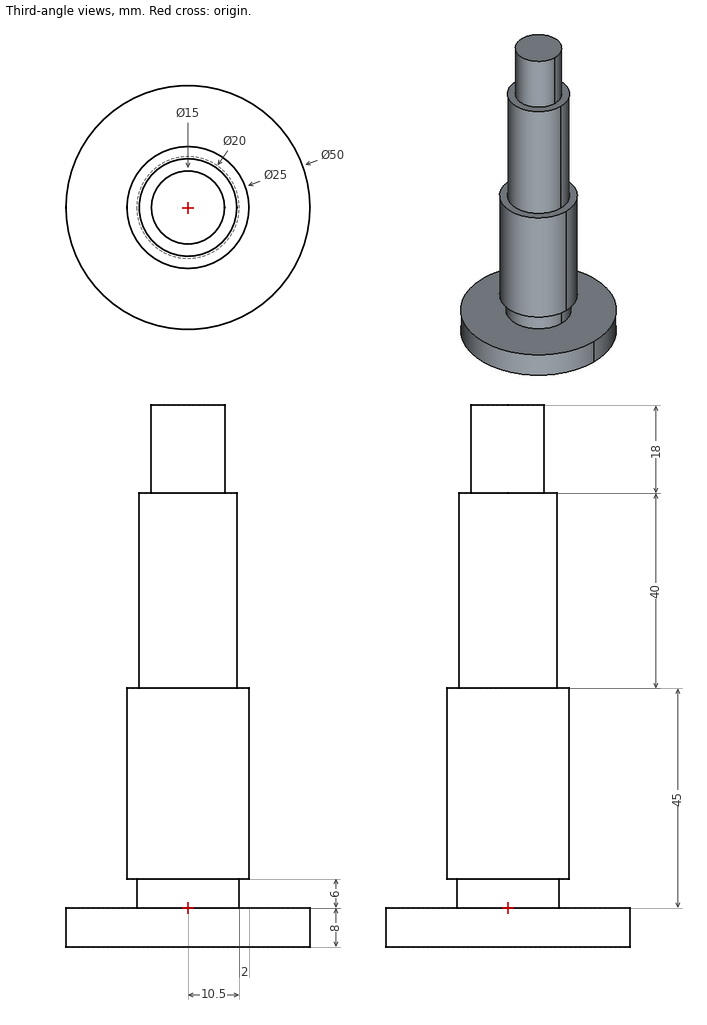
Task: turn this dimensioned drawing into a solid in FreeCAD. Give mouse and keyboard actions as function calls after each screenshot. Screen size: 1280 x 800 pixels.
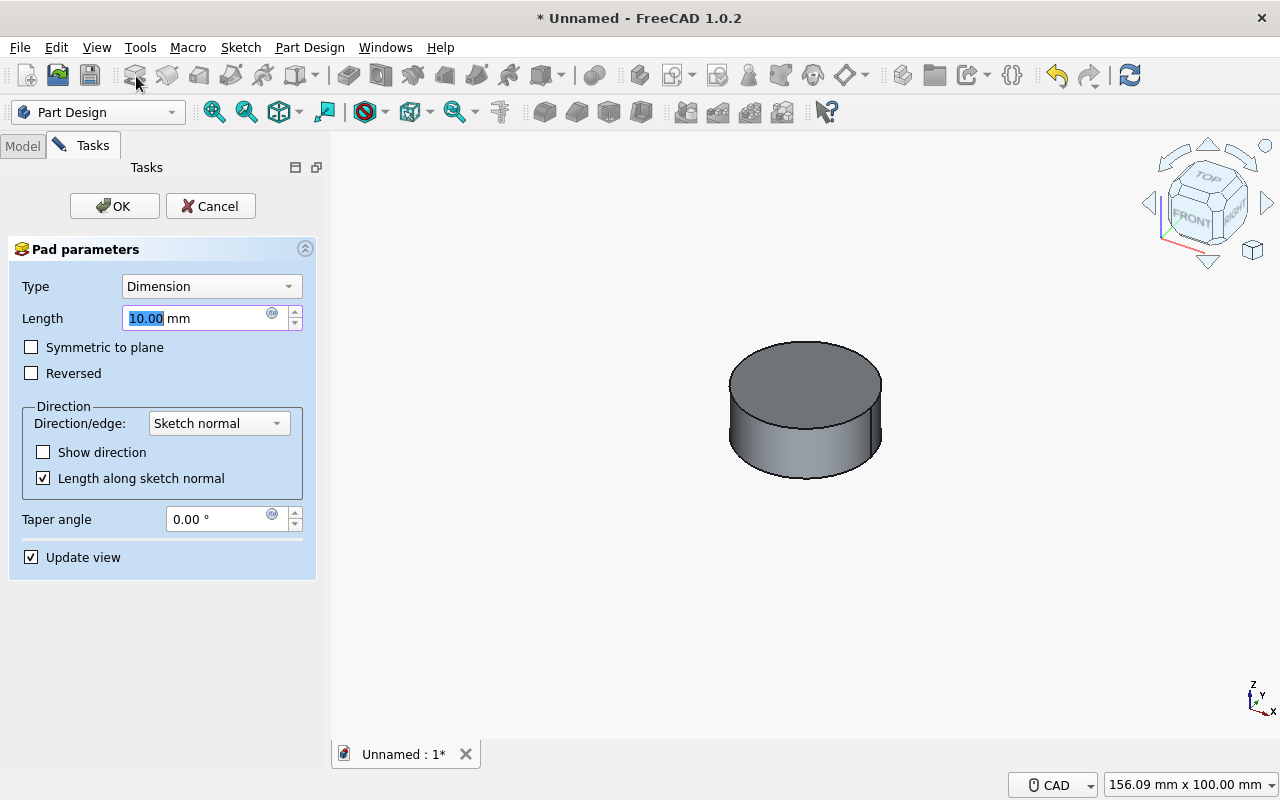
text(45)
key(Tab)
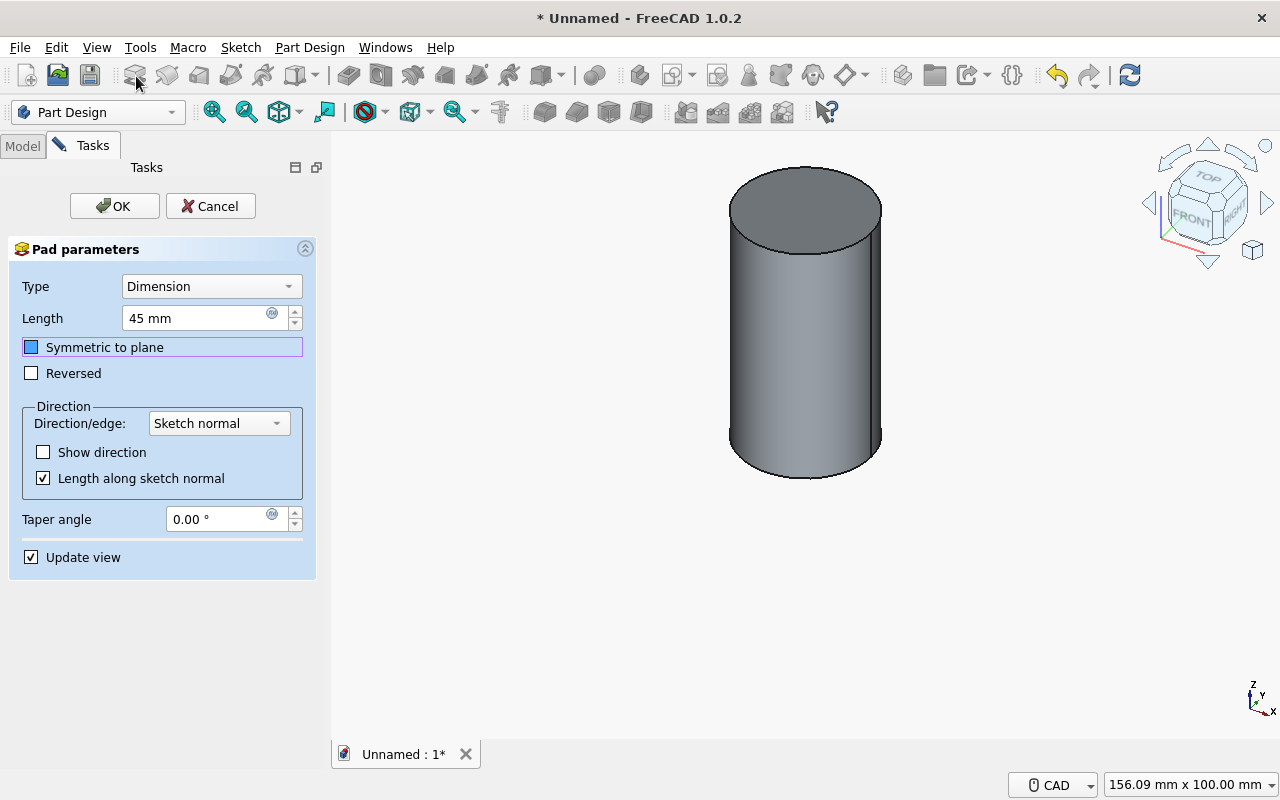
click(115, 206)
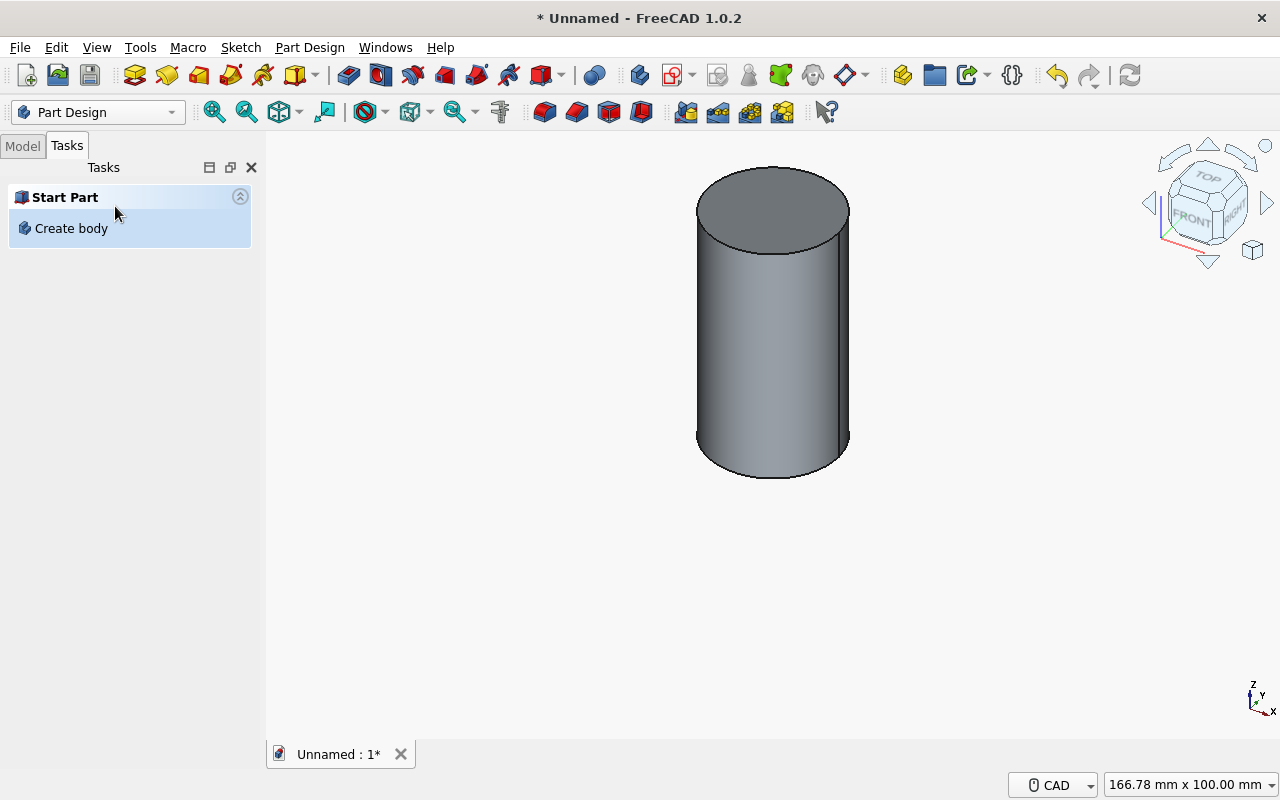
click(672, 76)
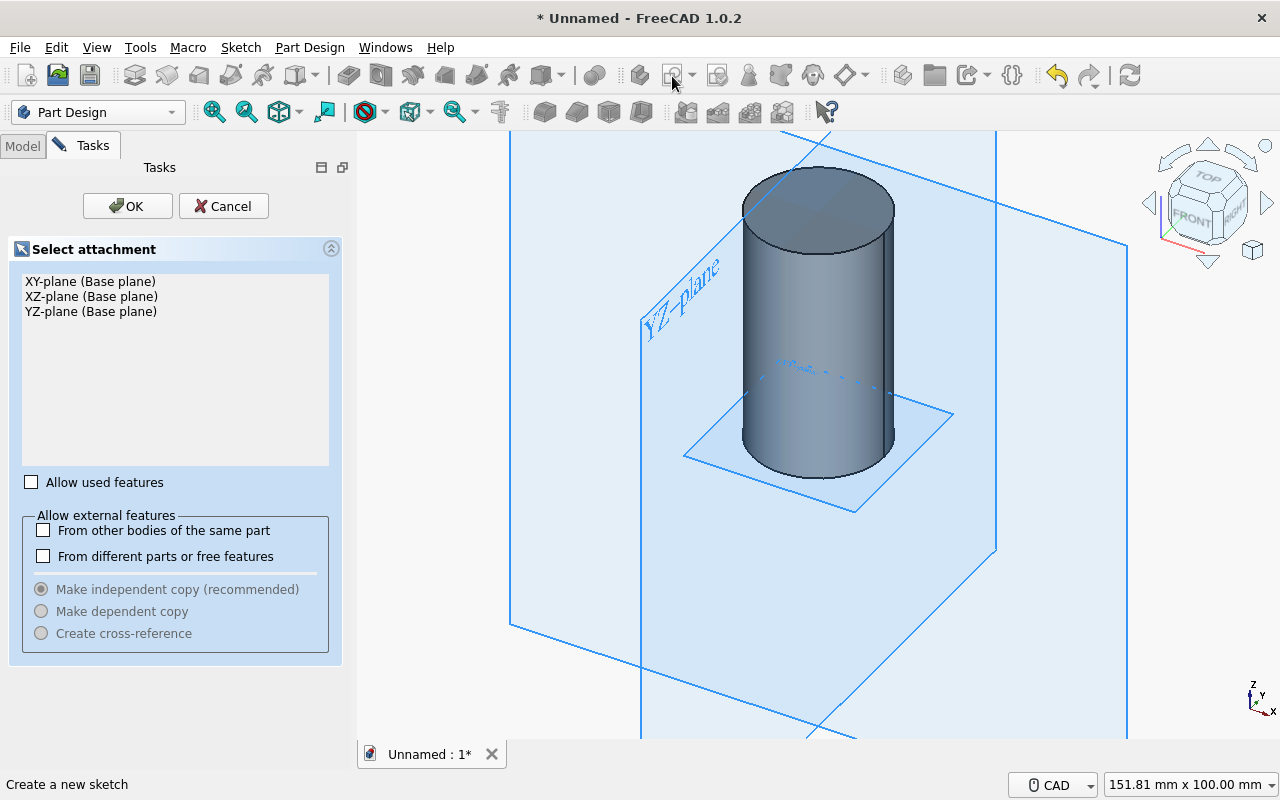
click(82, 282)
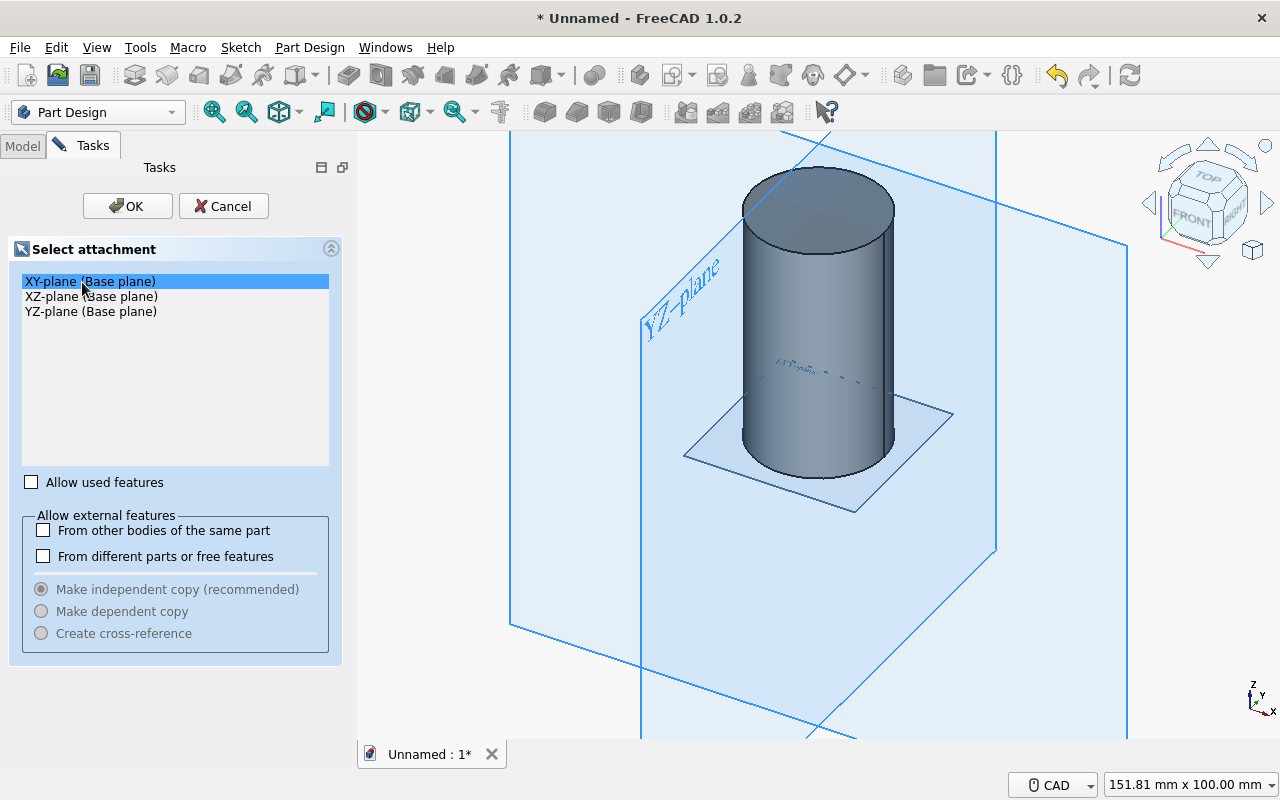
click(128, 206)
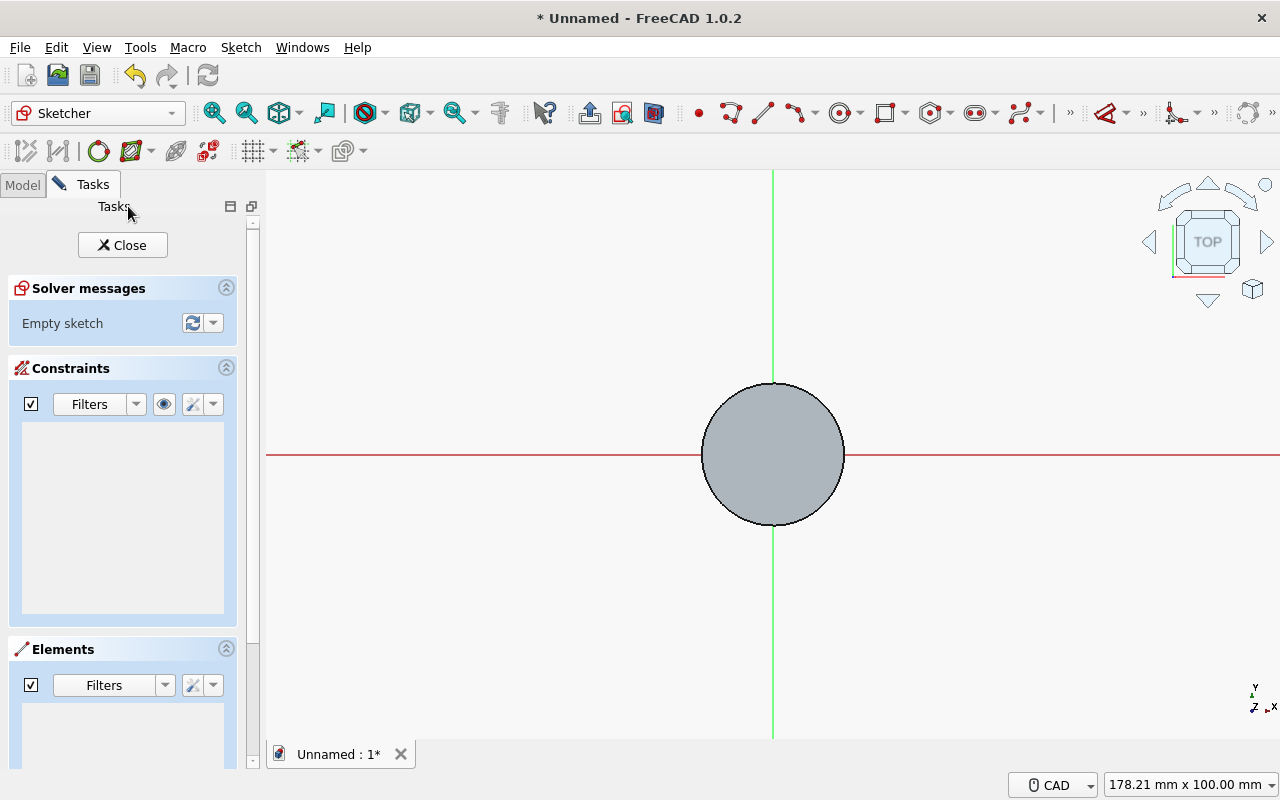
key(q)
key(s)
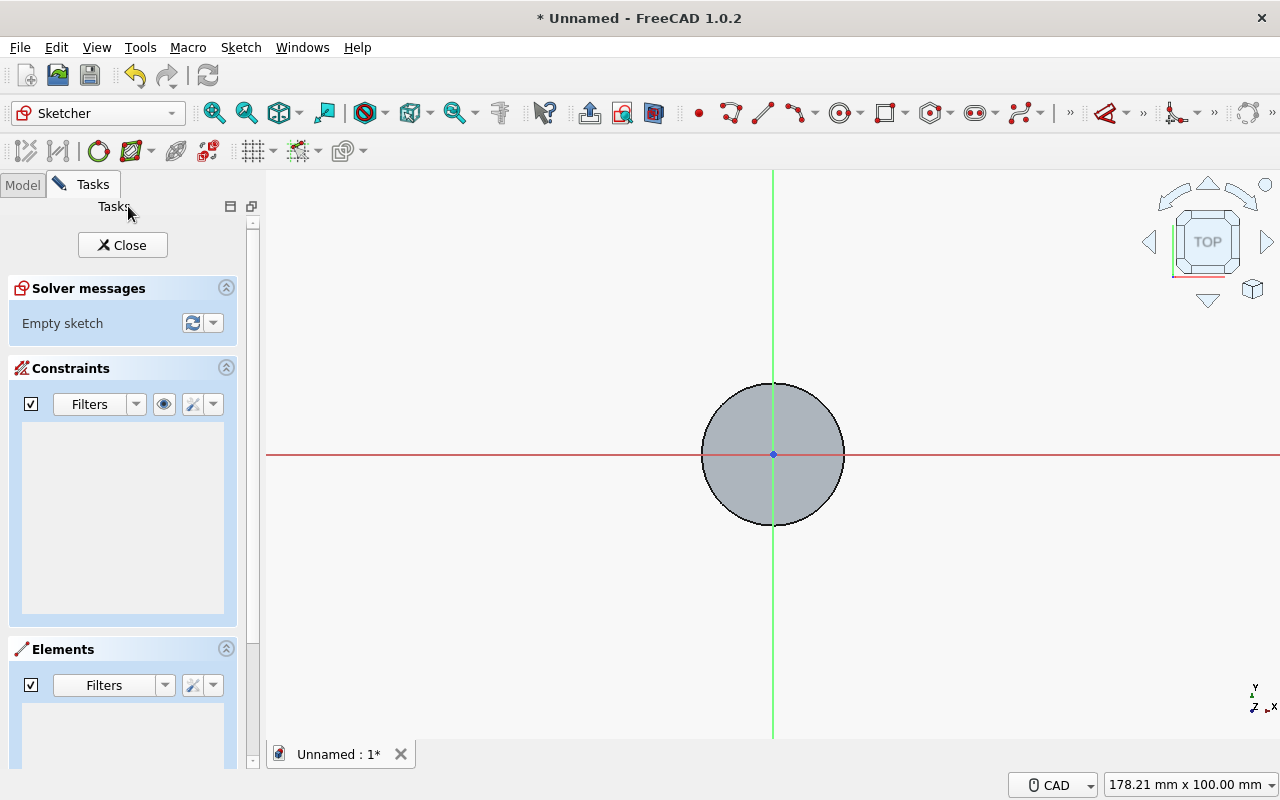
key(g)
key(c)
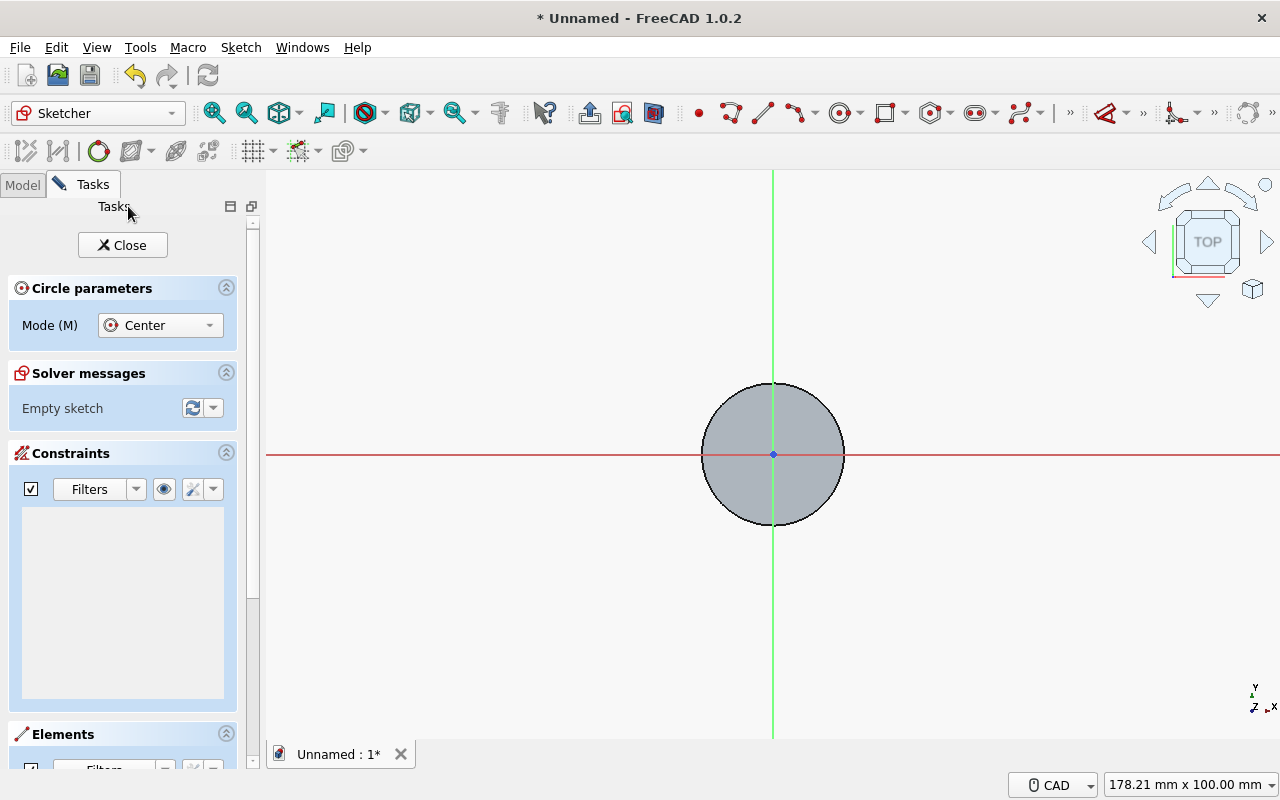
click(773, 454)
move(874, 354)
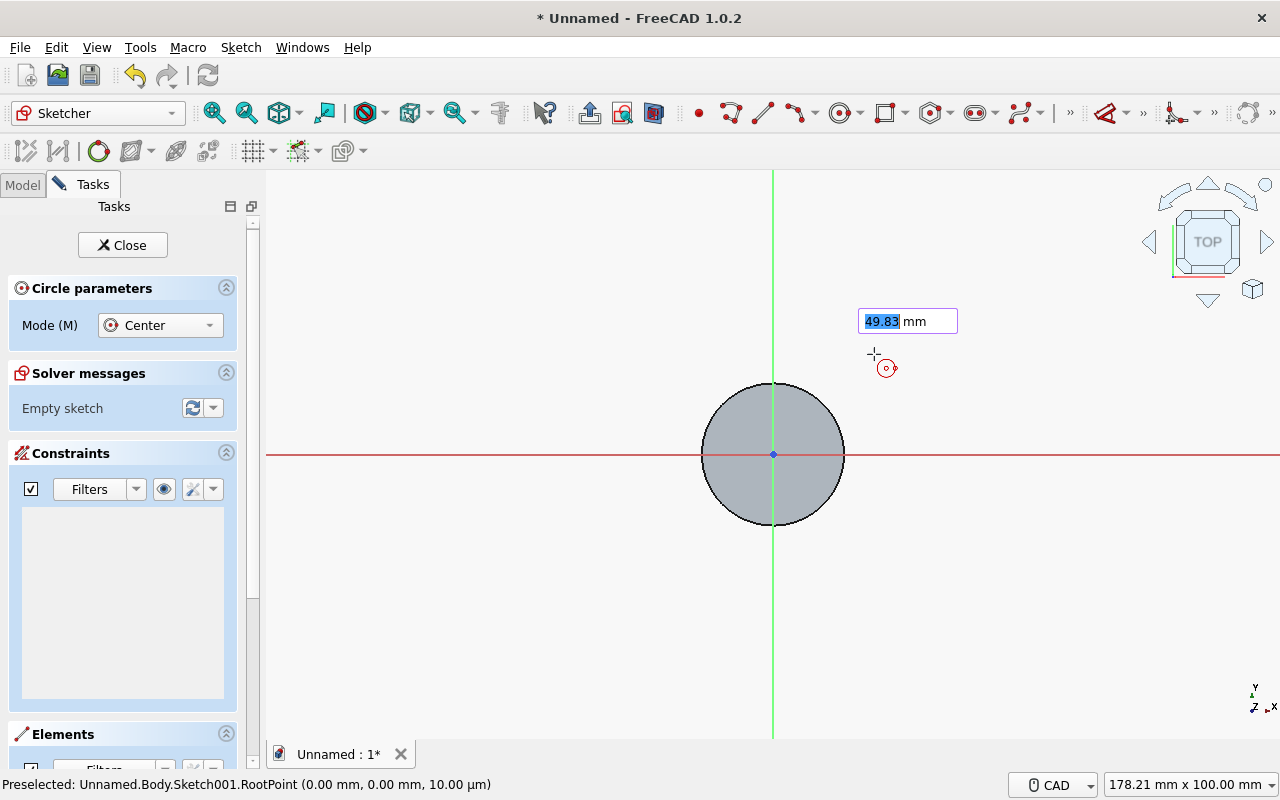
text(50)
key(Return)
key(Escape)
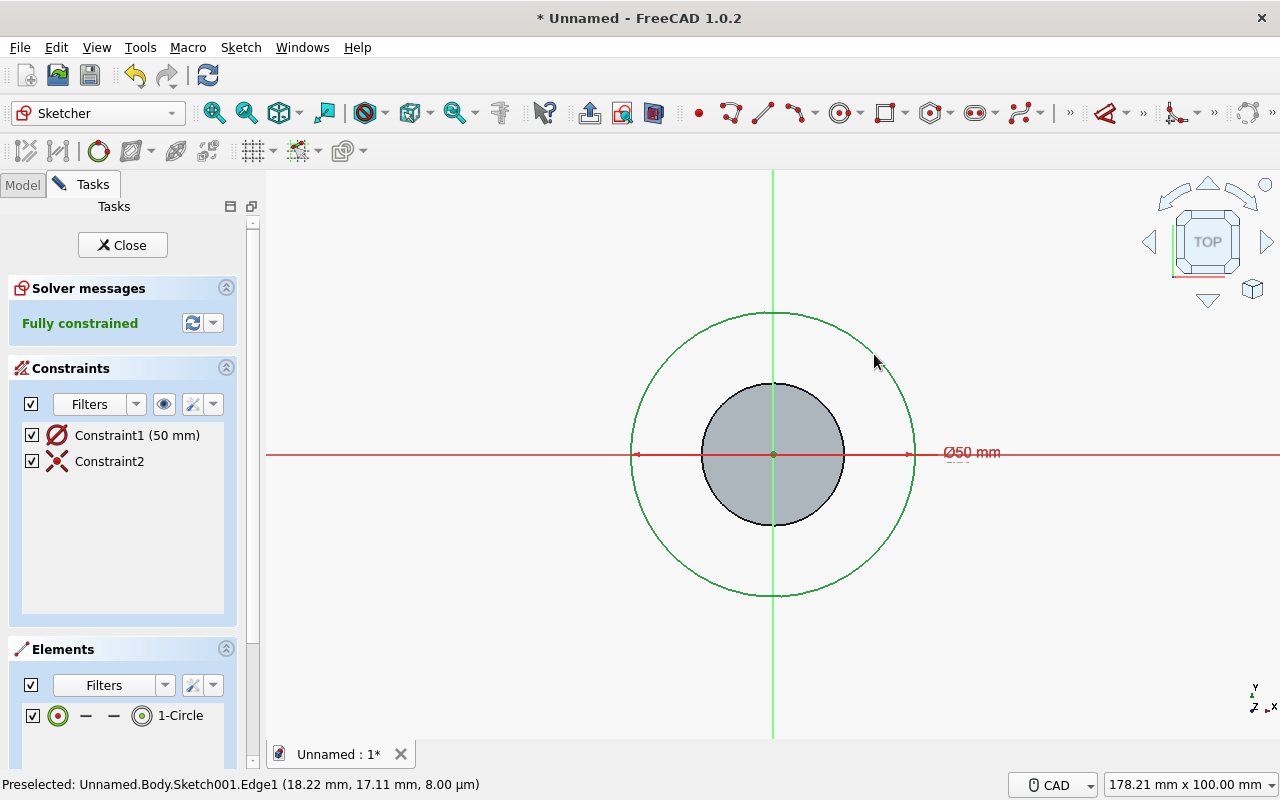
click(123, 245)